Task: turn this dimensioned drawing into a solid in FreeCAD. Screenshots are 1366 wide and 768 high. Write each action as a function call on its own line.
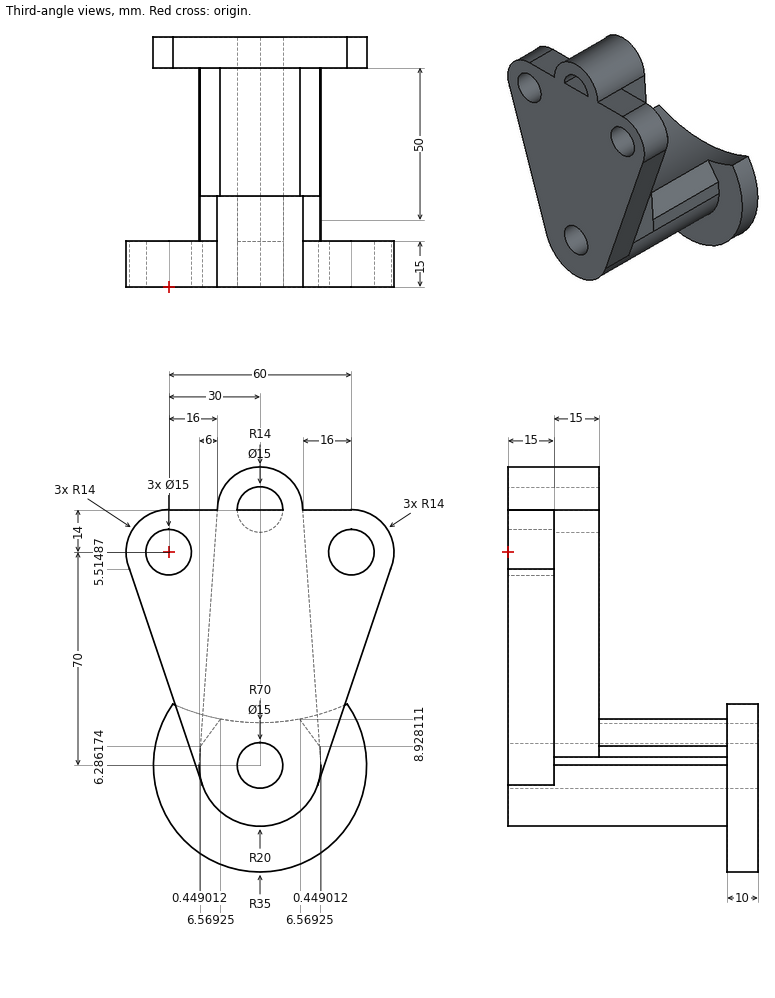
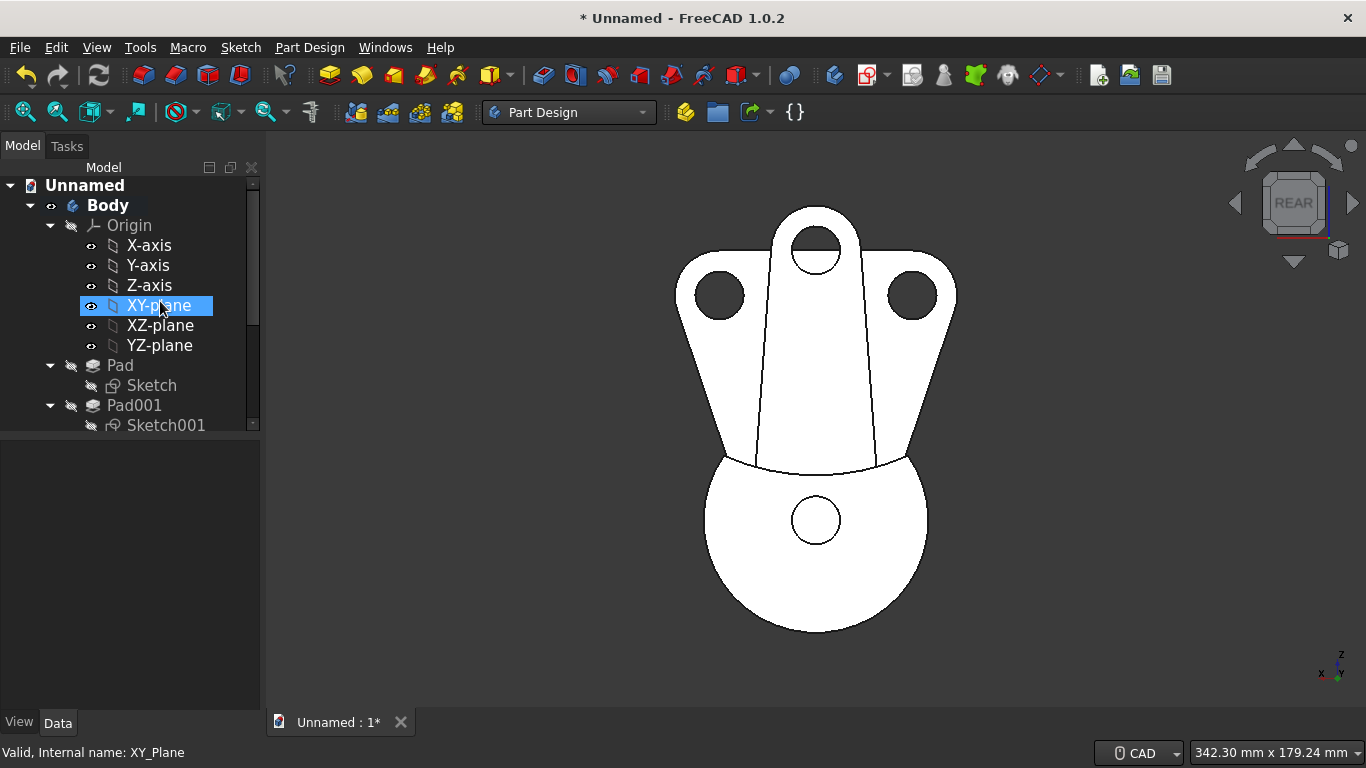
click(136, 326)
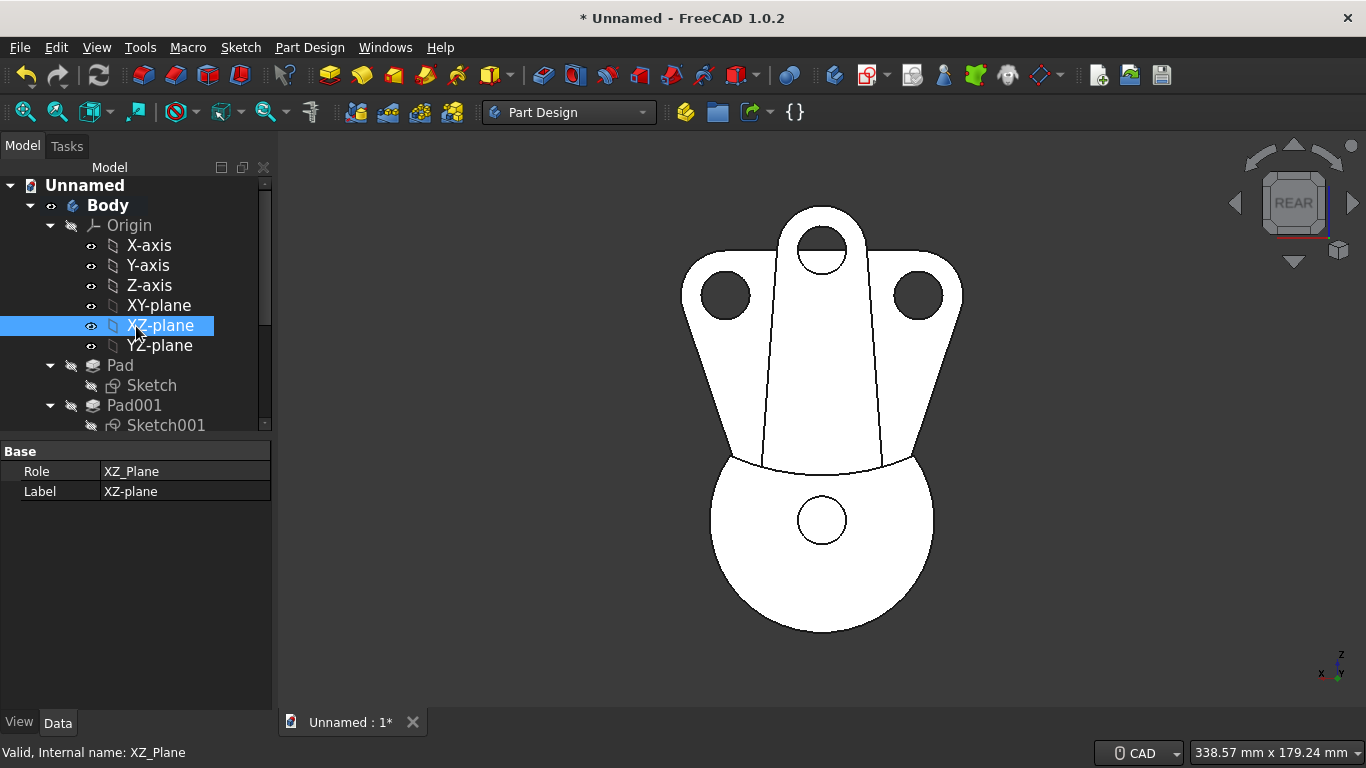
click(1040, 76)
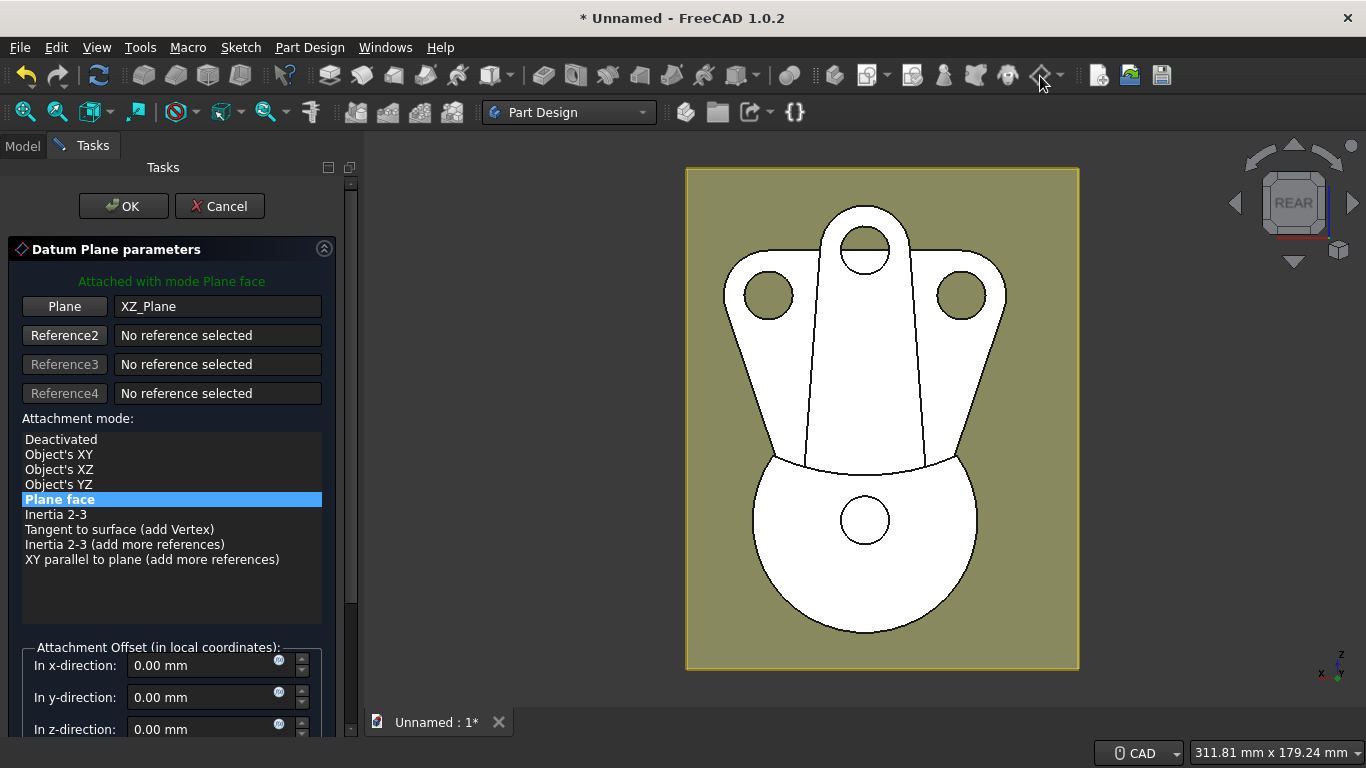
scroll(351, 456, down, 2)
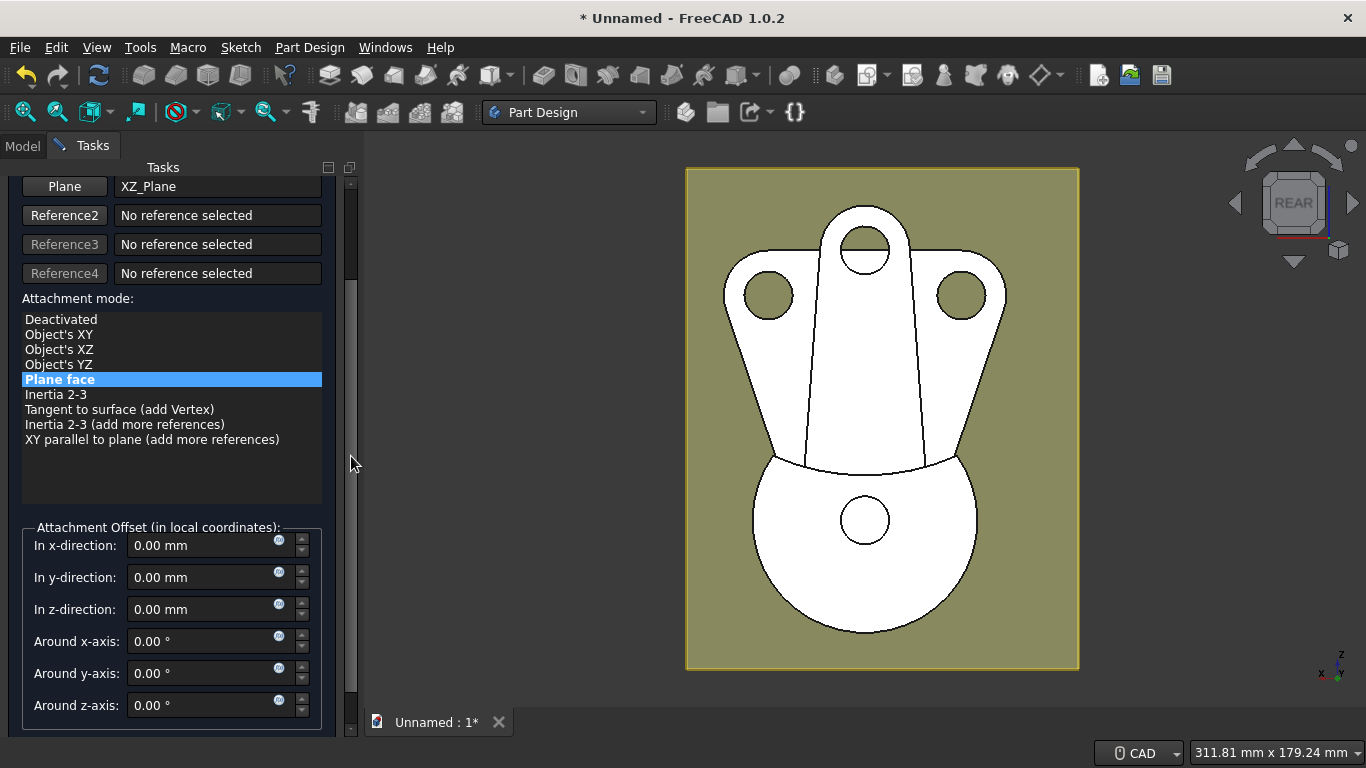
triple_click(210, 609)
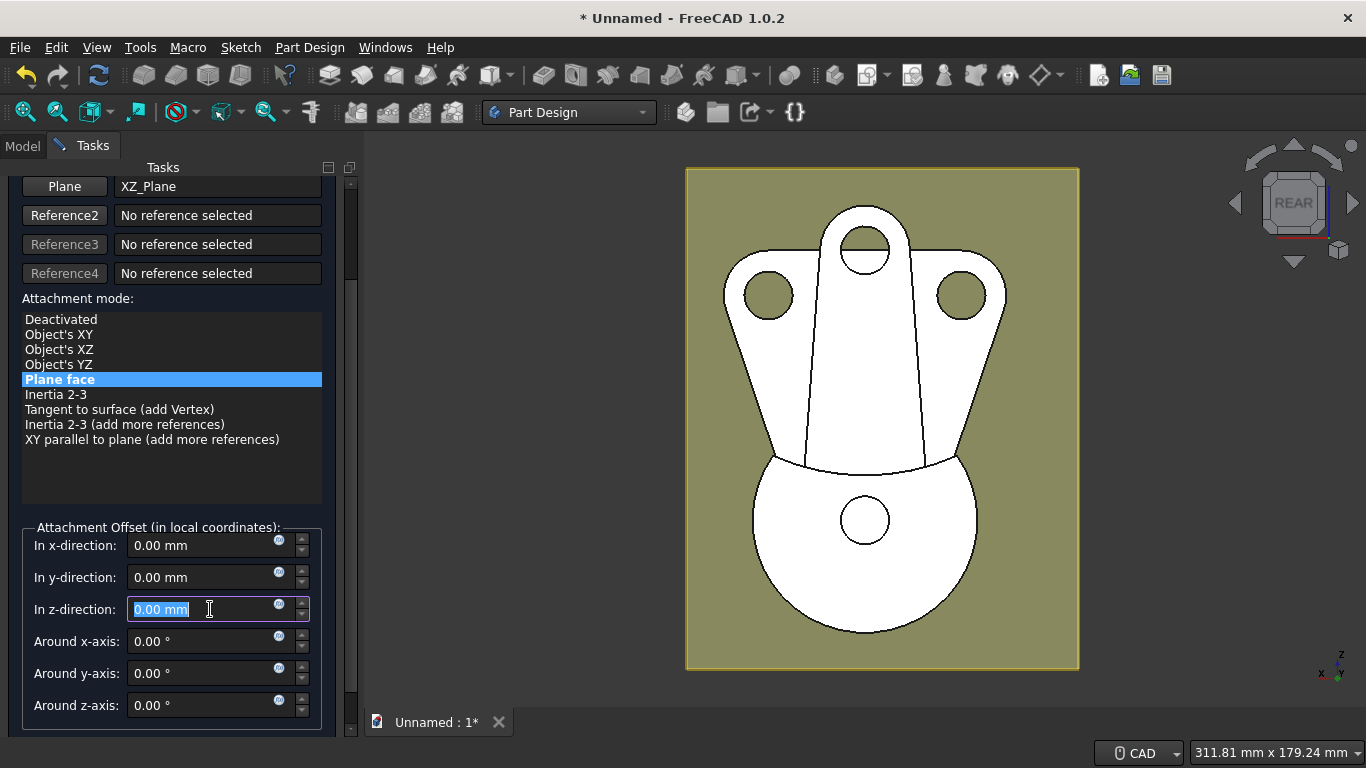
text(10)
key(Tab)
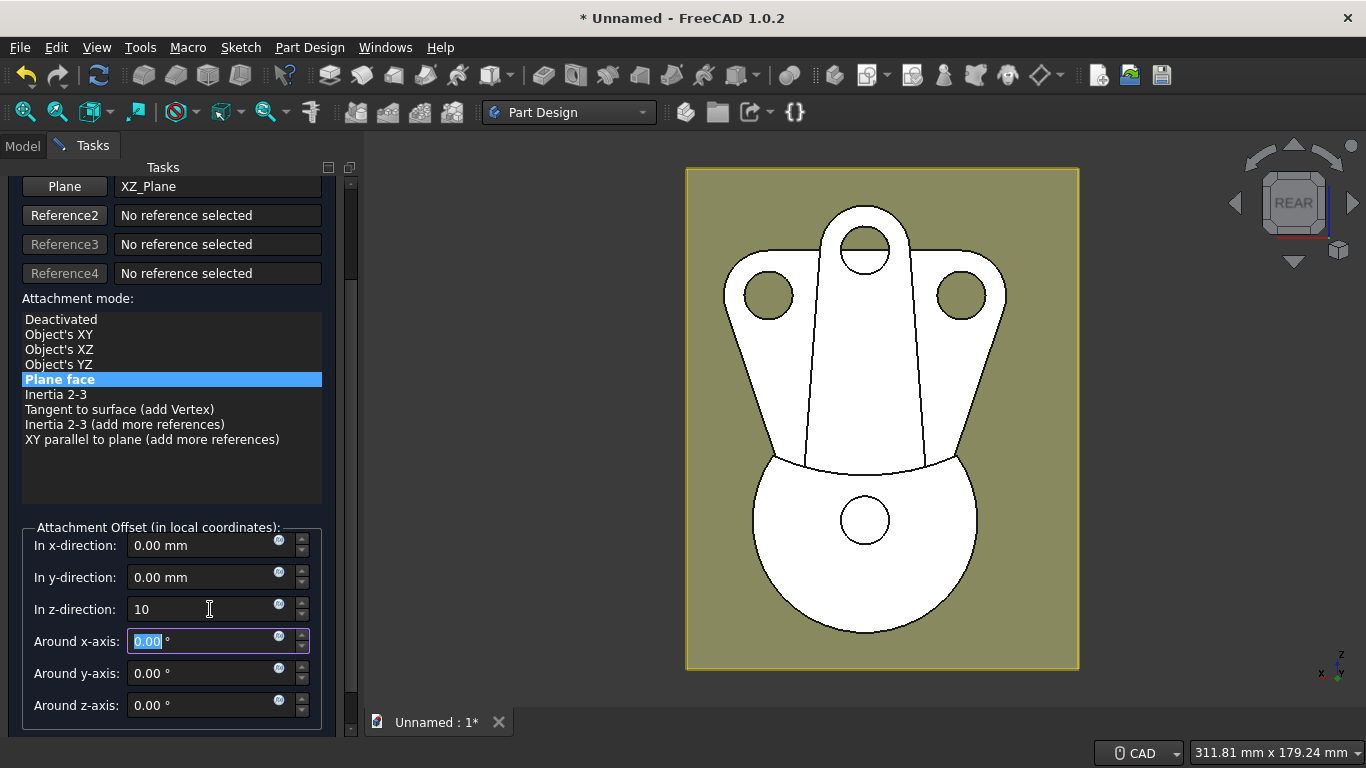
scroll(351, 456, up, 3)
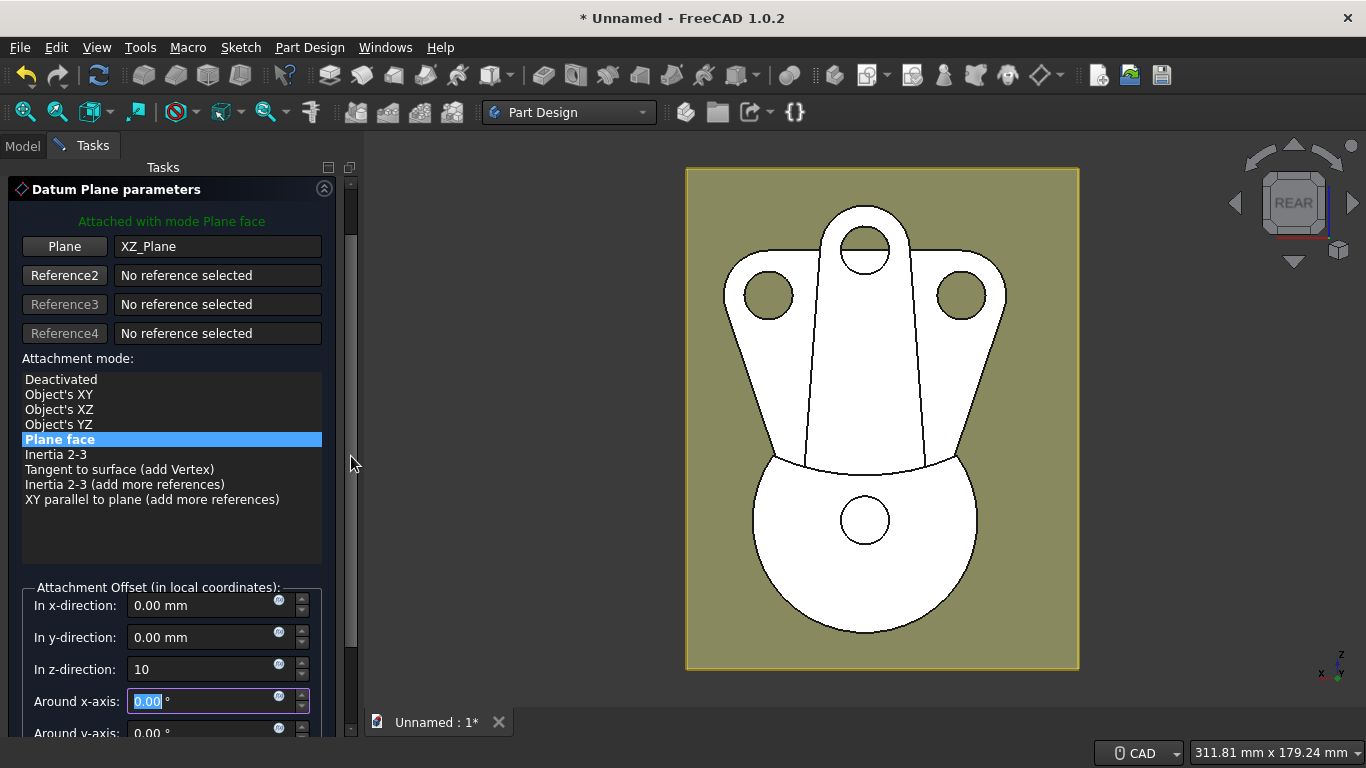
click(124, 206)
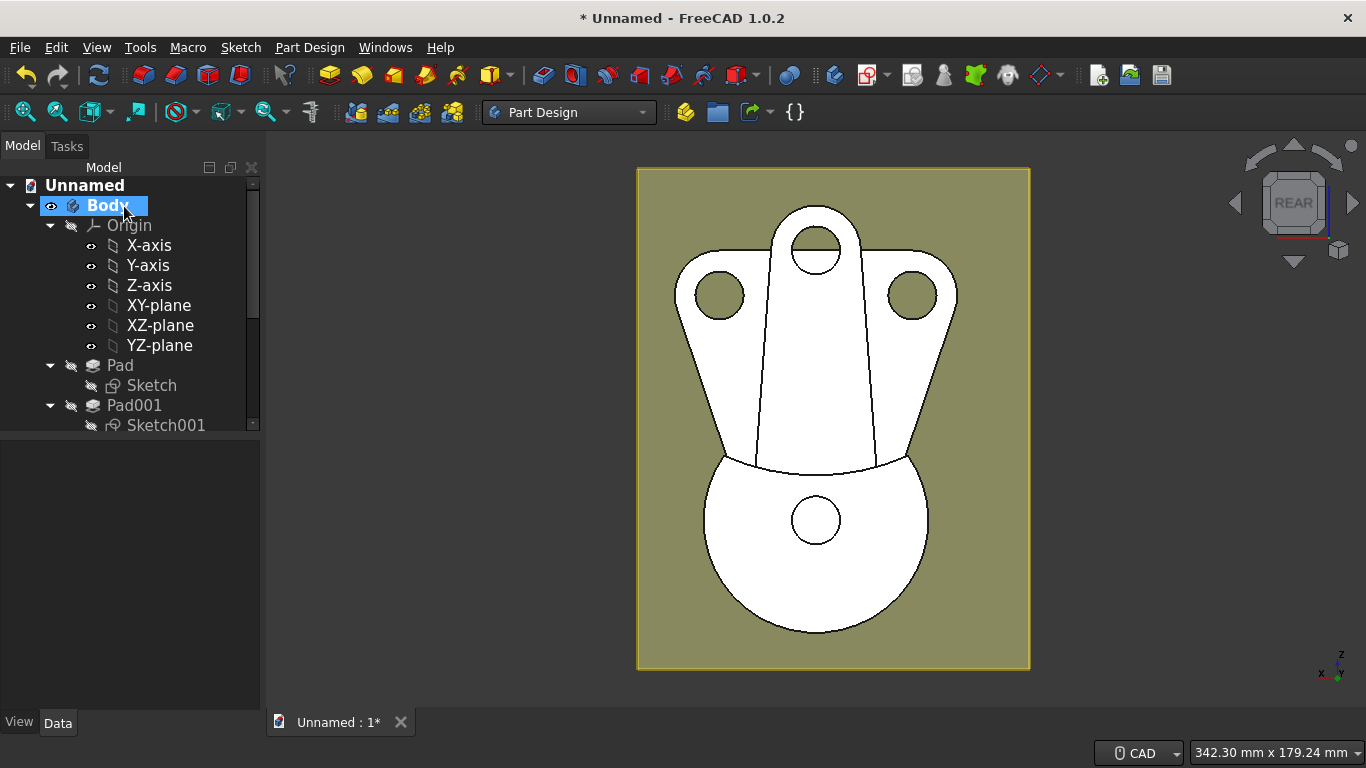
scroll(100, 301, down, 3)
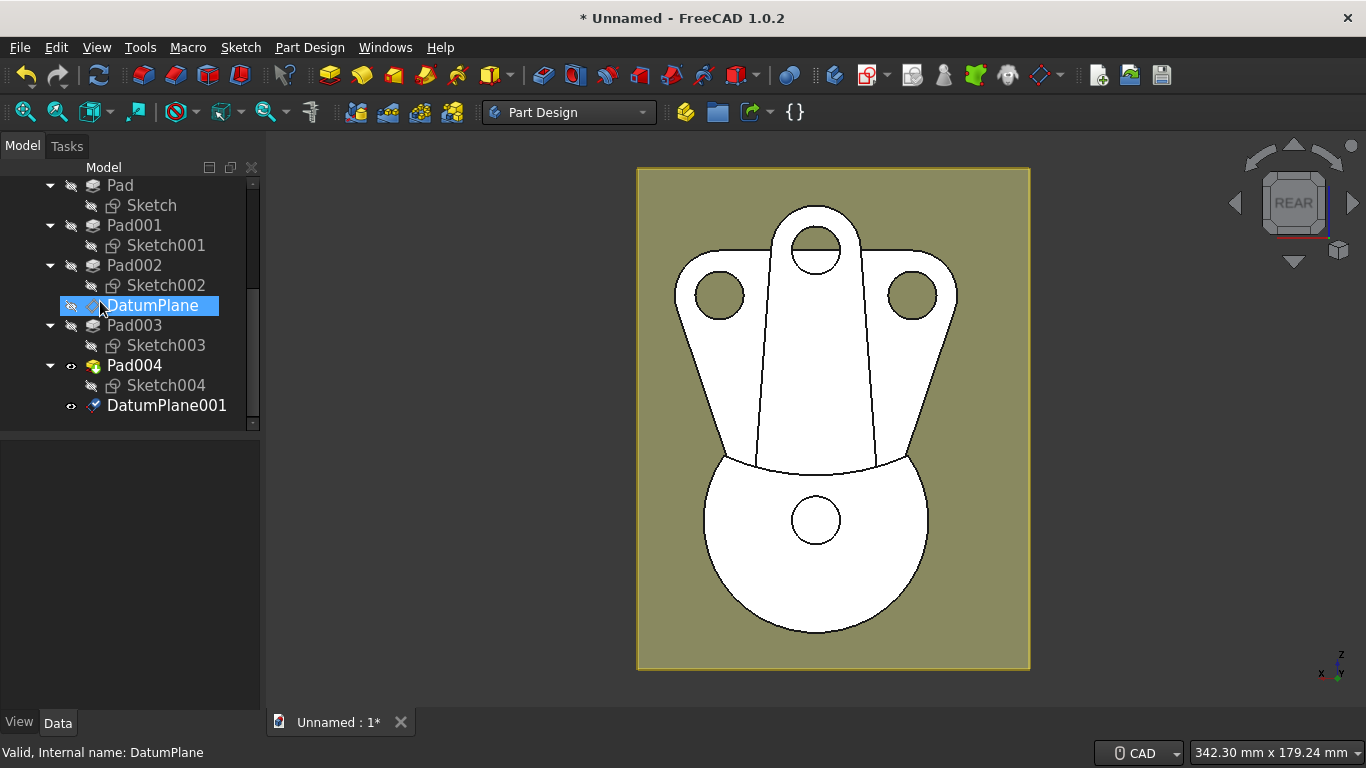
click(116, 406)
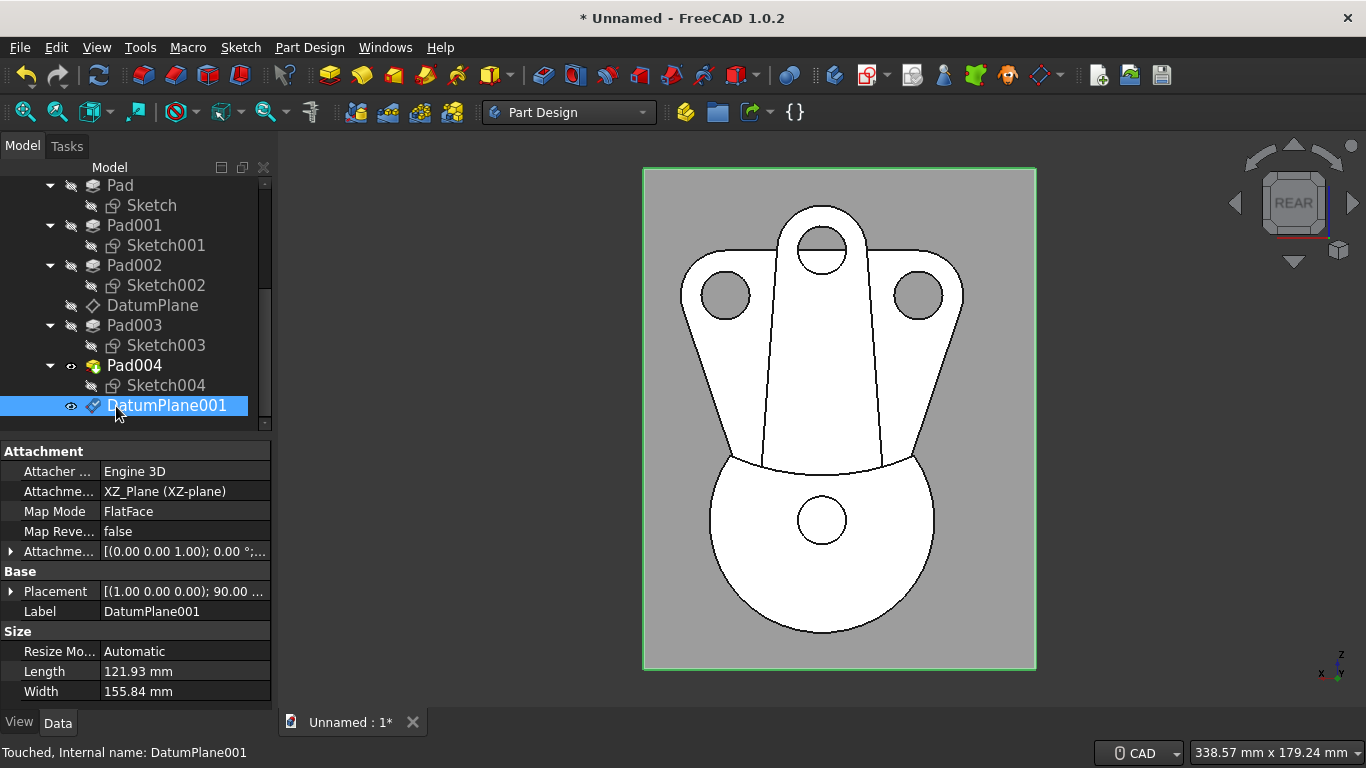
click(868, 76)